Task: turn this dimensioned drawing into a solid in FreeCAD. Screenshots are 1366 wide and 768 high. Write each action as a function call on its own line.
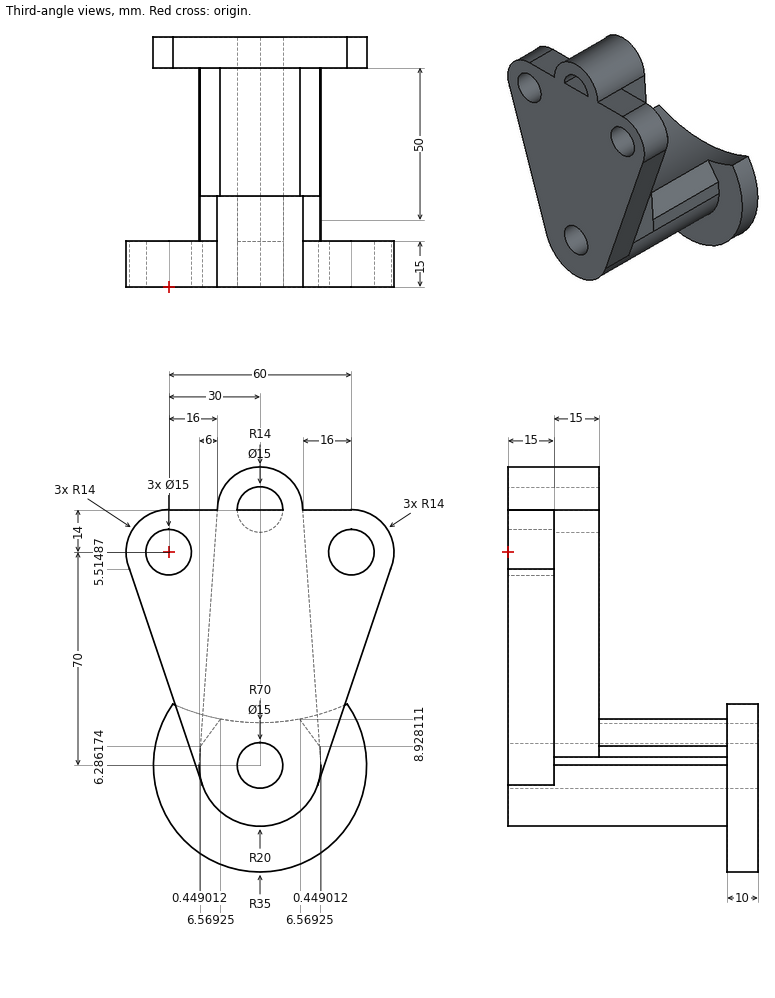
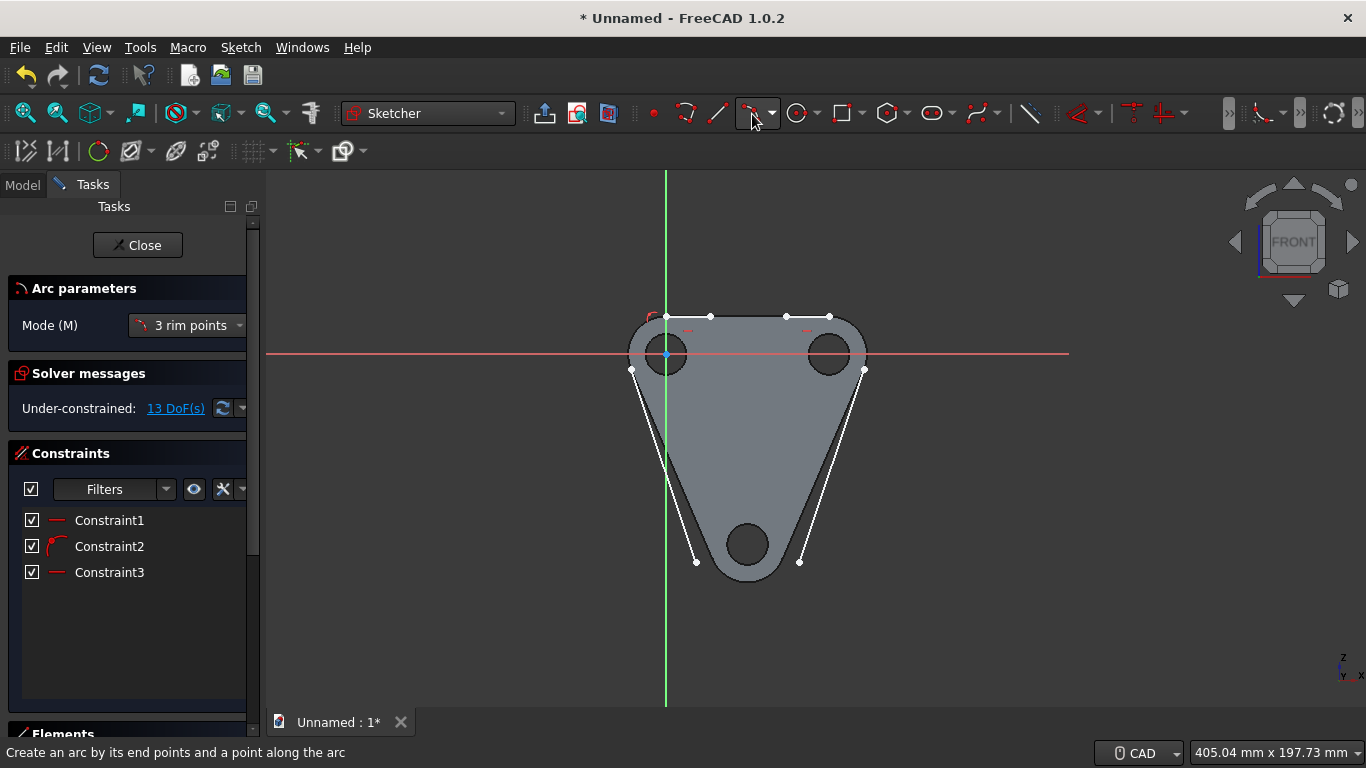
click(696, 563)
click(799, 563)
click(748, 599)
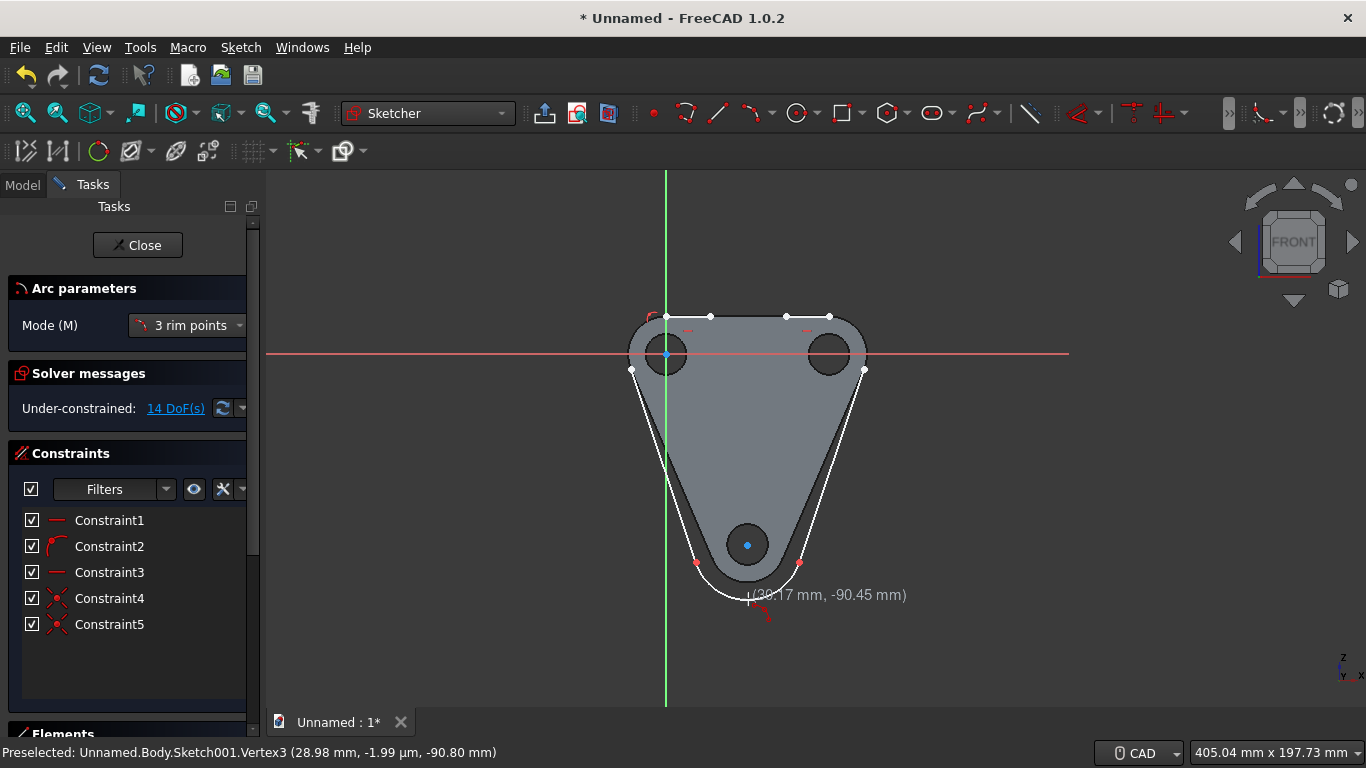
click(864, 370)
click(829, 317)
click(861, 333)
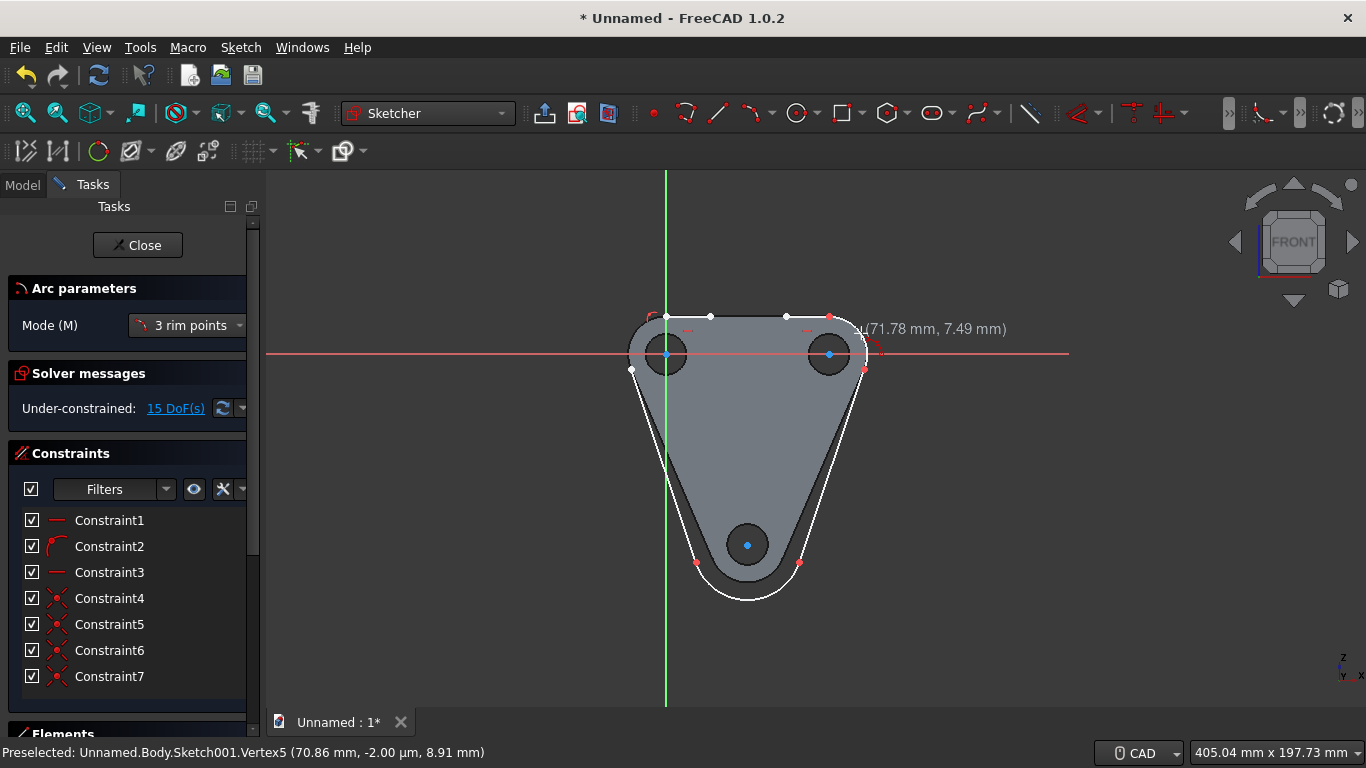
click(786, 317)
click(710, 317)
click(748, 278)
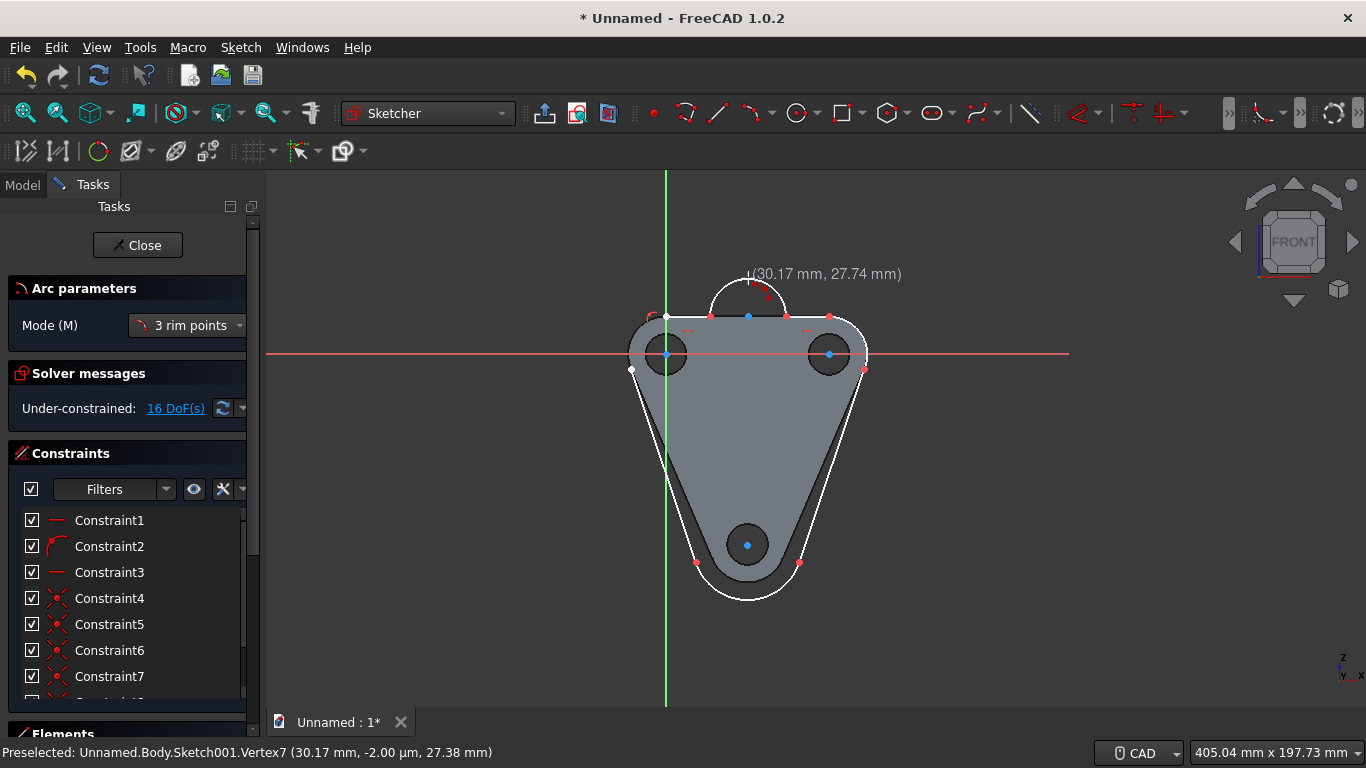
click(666, 317)
click(631, 370)
click(634, 333)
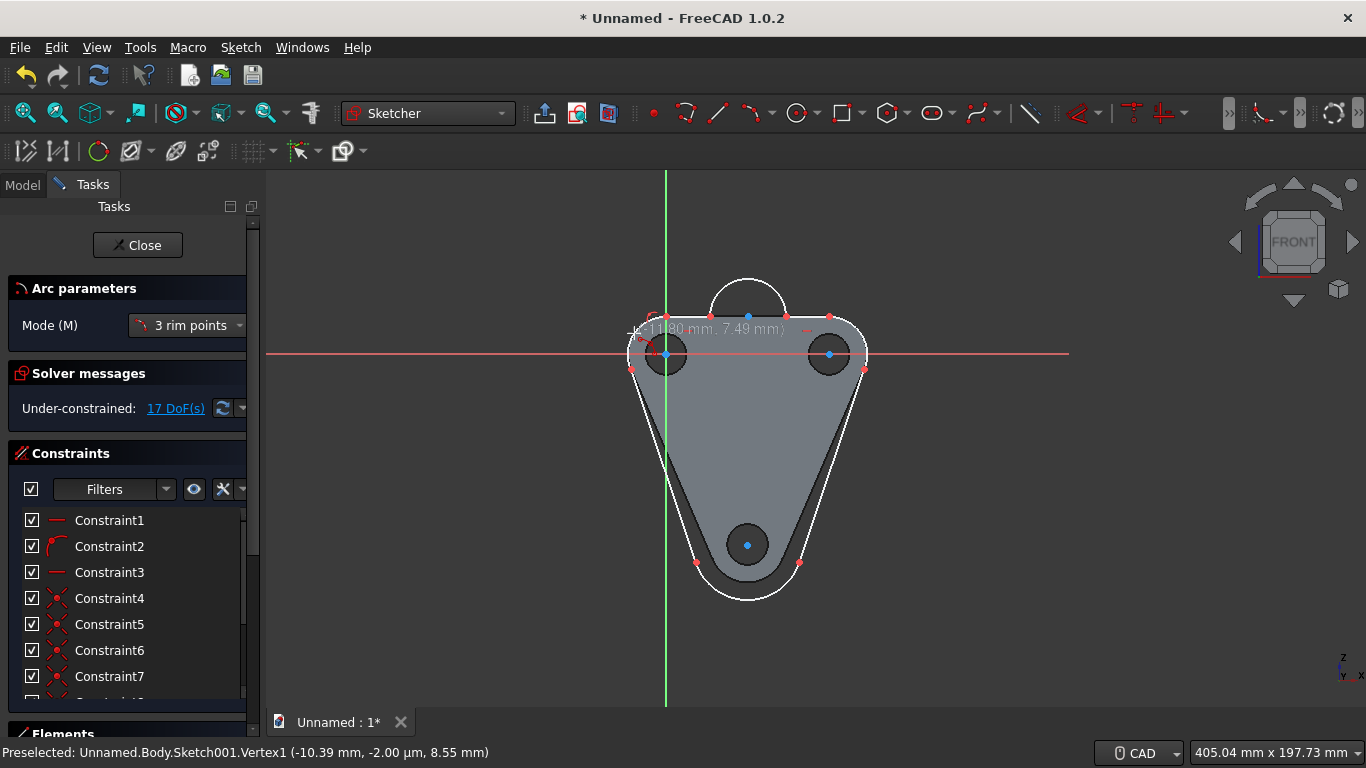
click(798, 114)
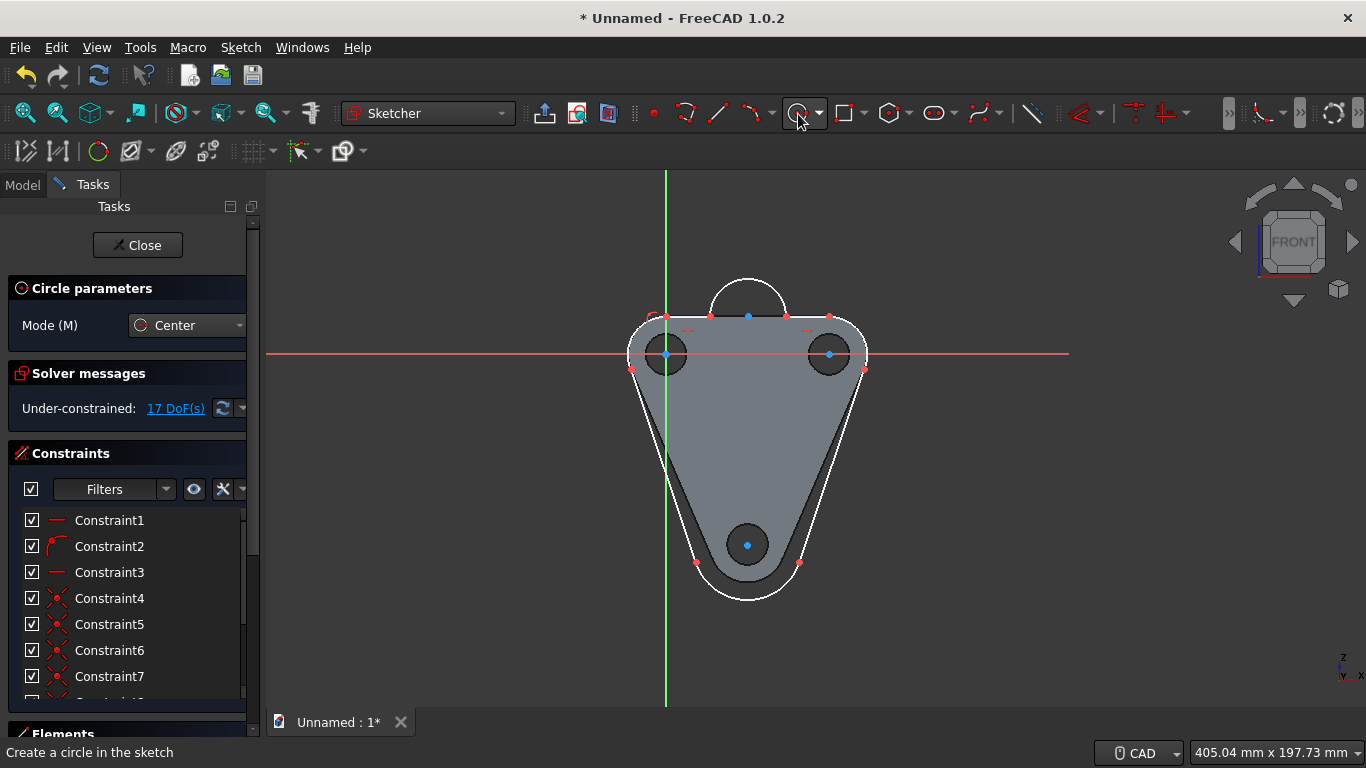
click(666, 354)
move(680, 340)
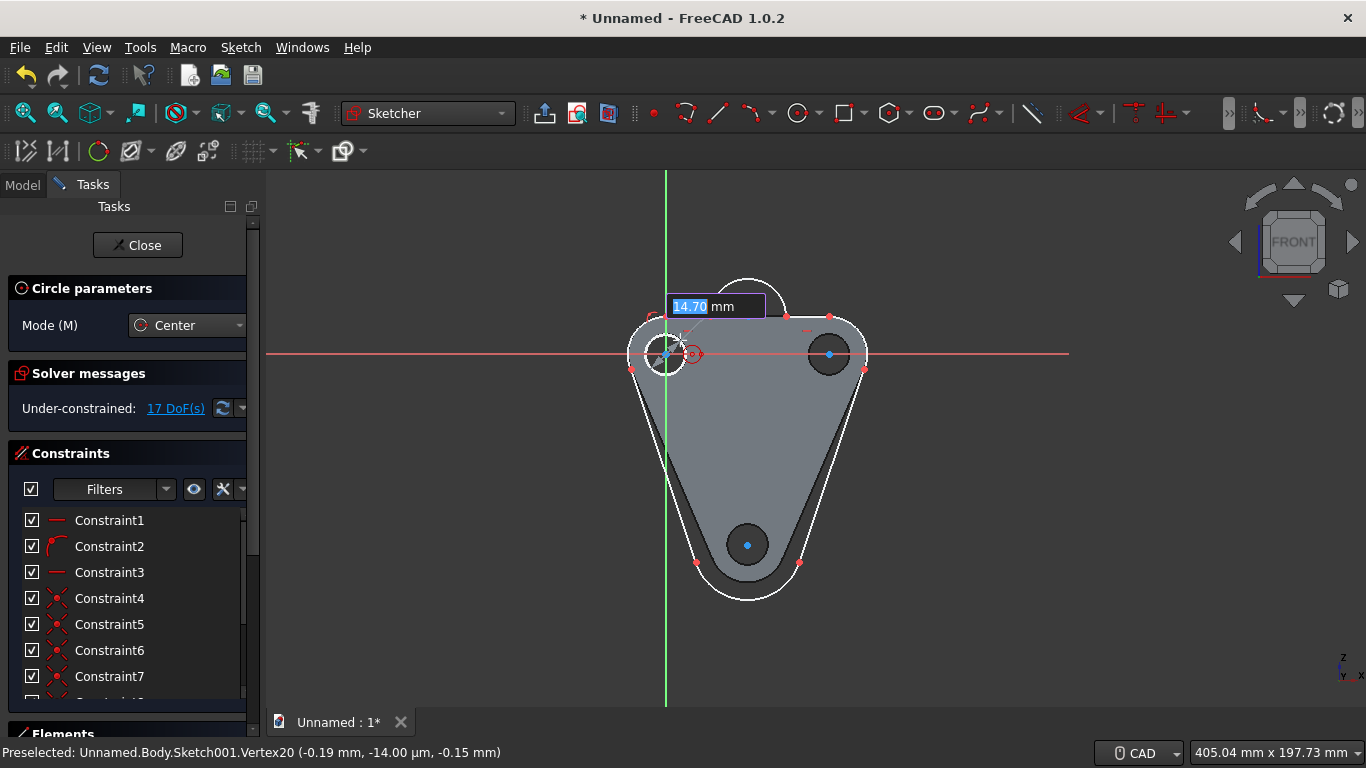
text(15)
key(Return)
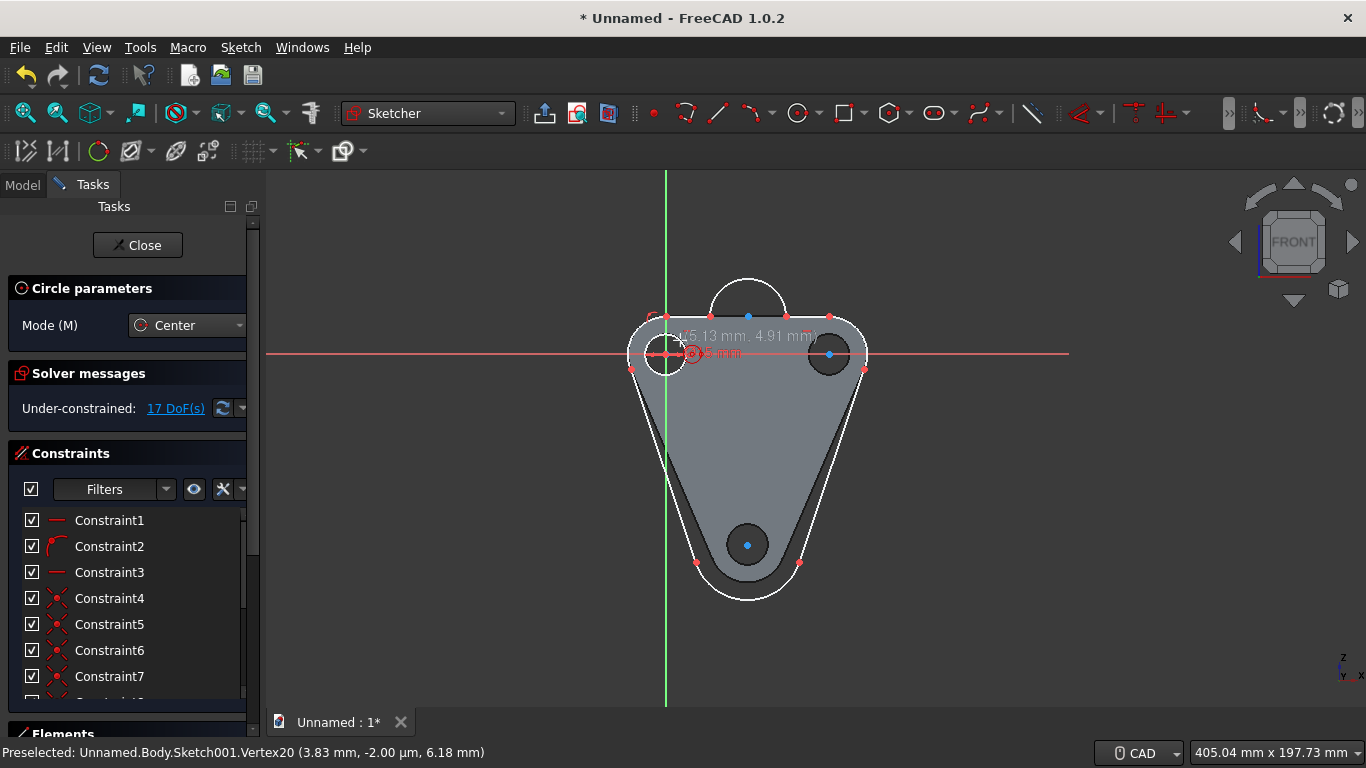
click(829, 354)
move(843, 340)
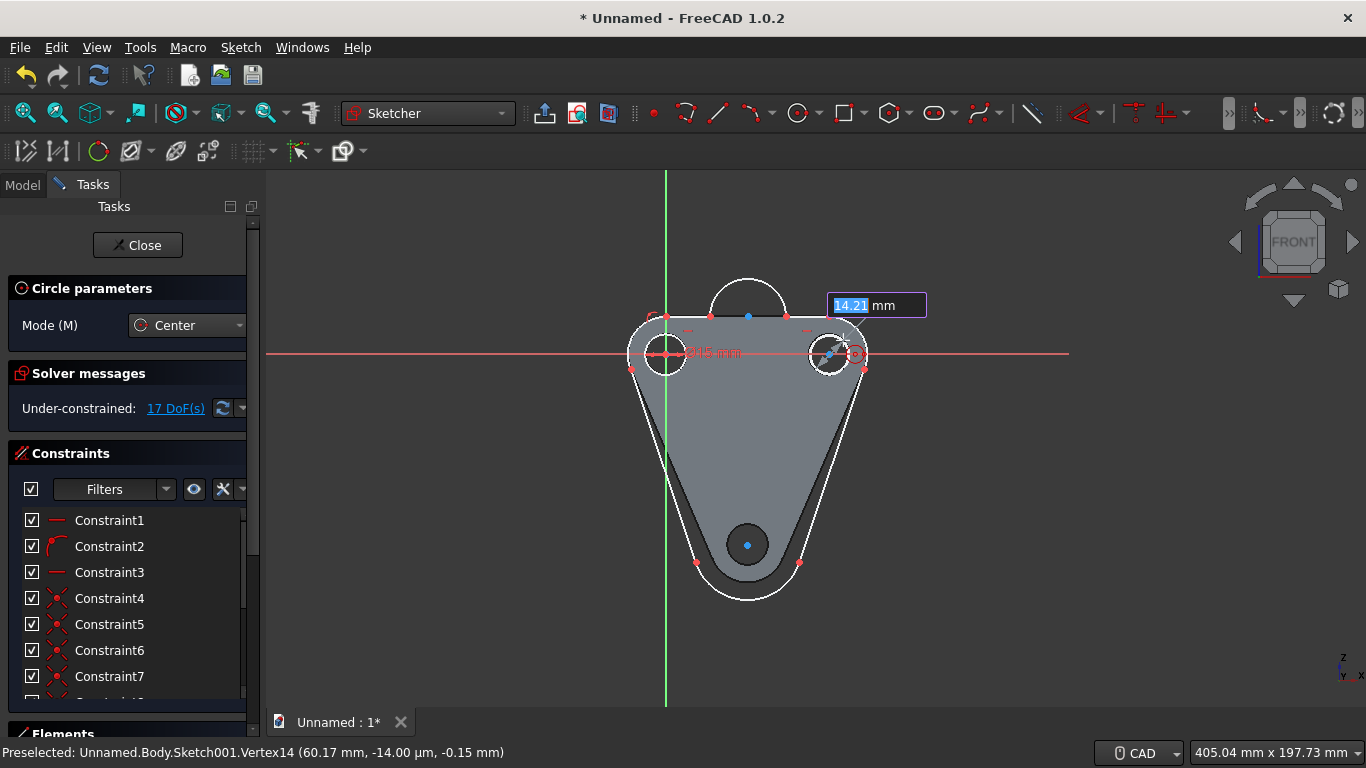
text(15)
key(Return)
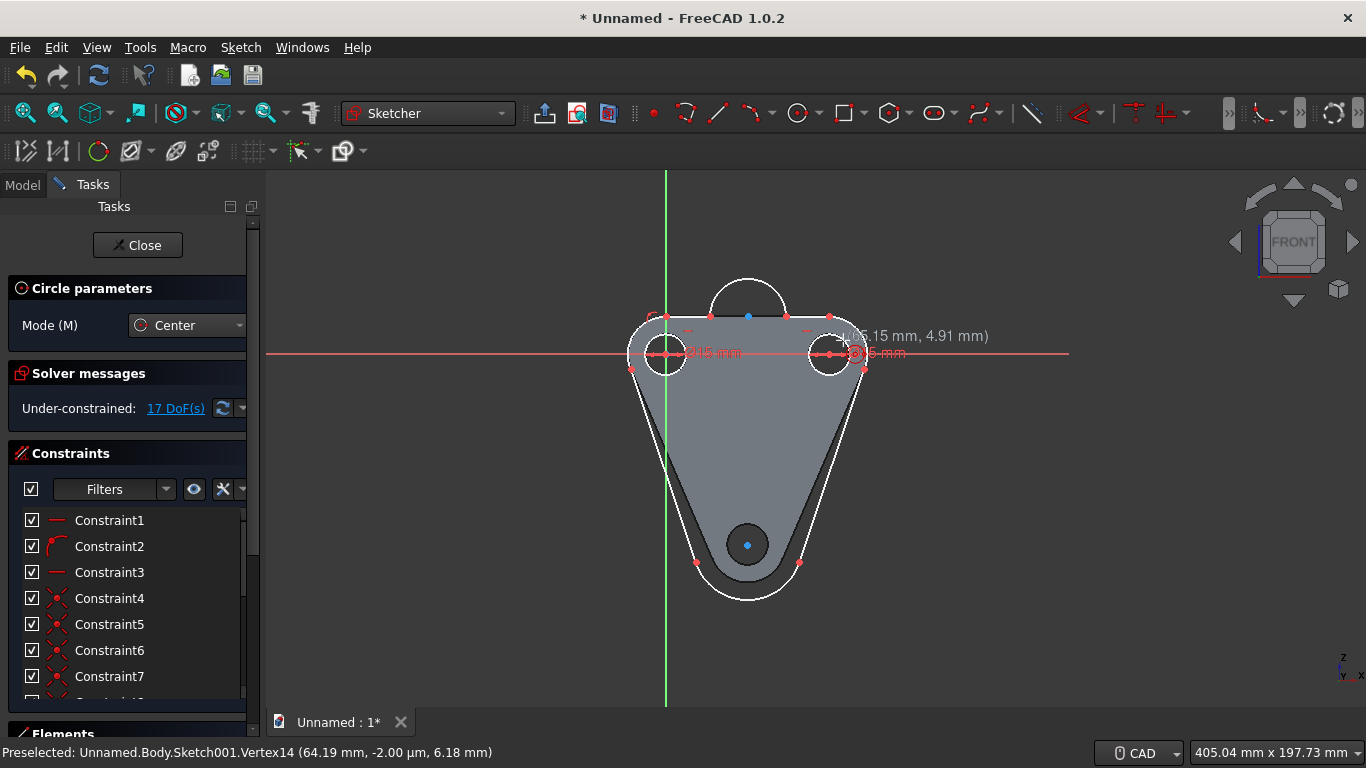
click(748, 316)
move(762, 302)